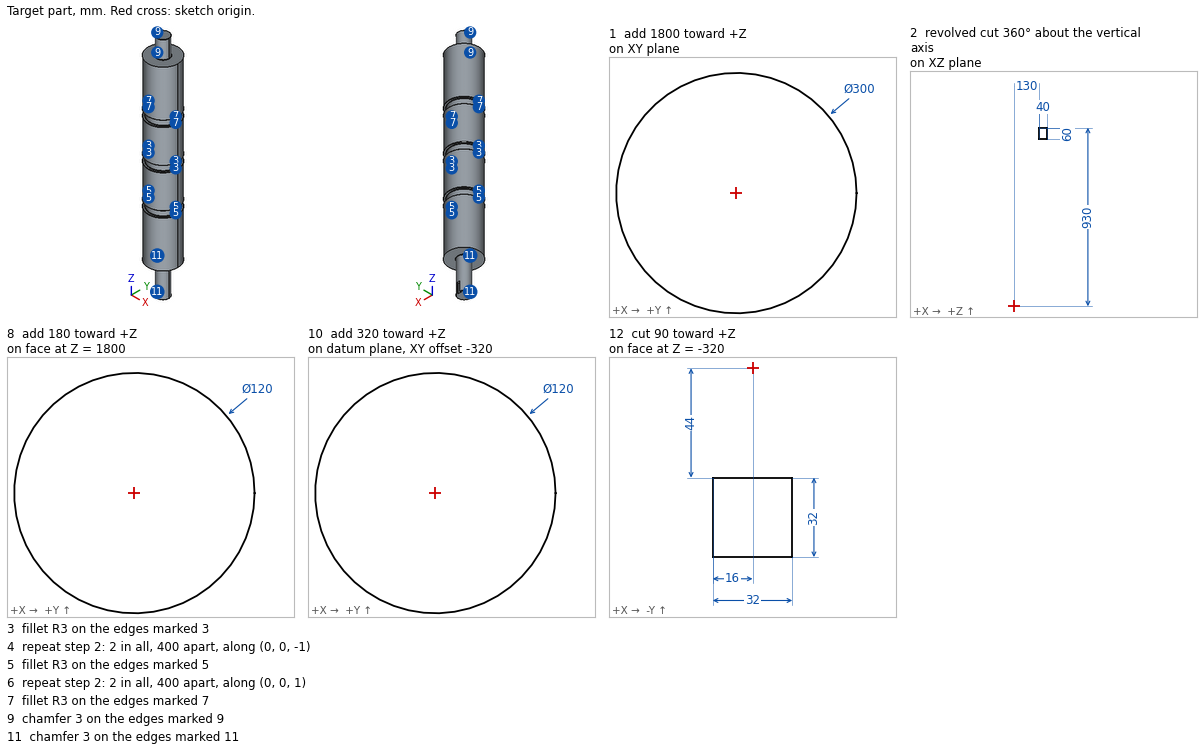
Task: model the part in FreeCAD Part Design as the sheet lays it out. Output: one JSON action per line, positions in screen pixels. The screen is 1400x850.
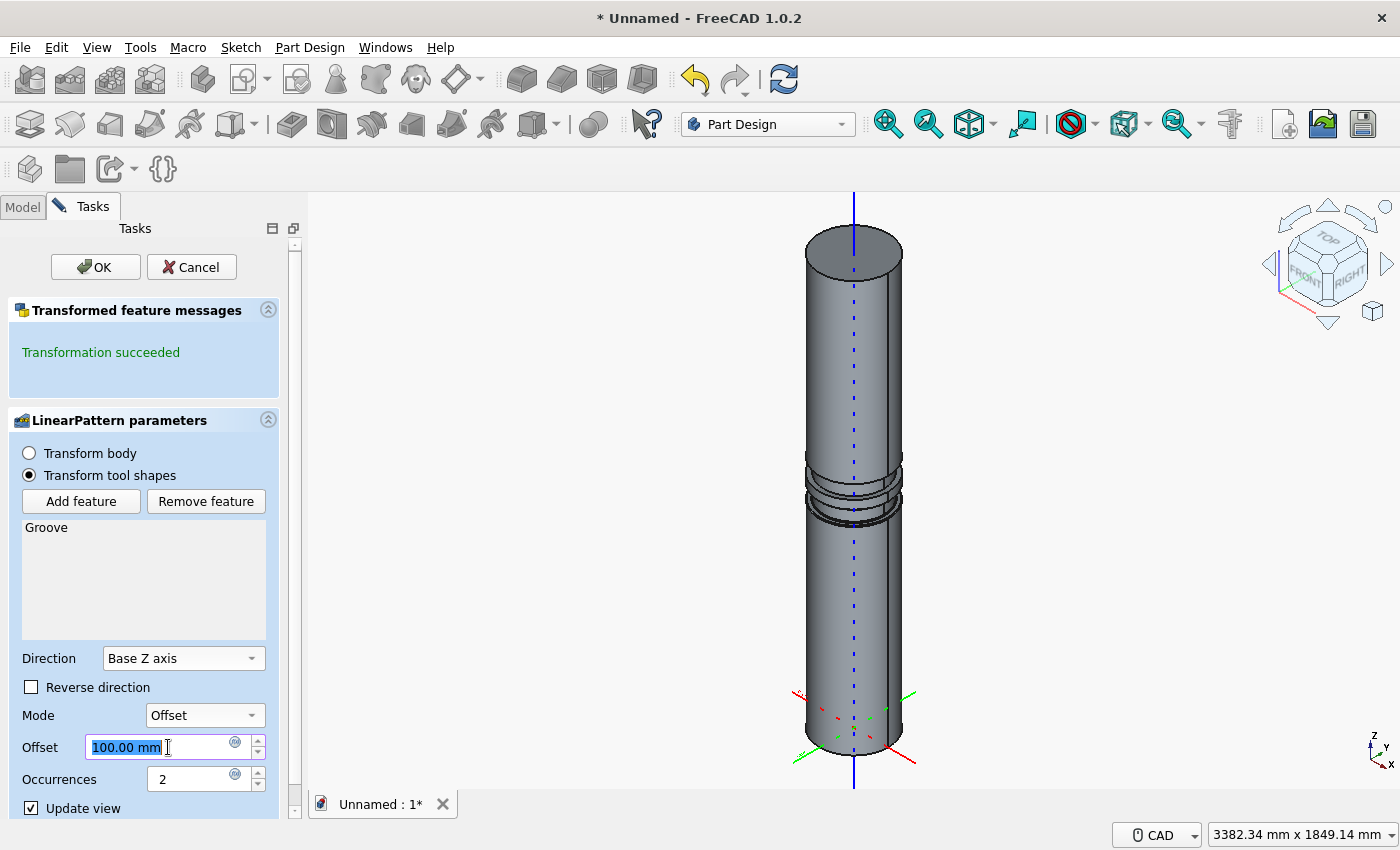
{"action": "type", "text": "400"}
{"action": "key", "text": "Tab"}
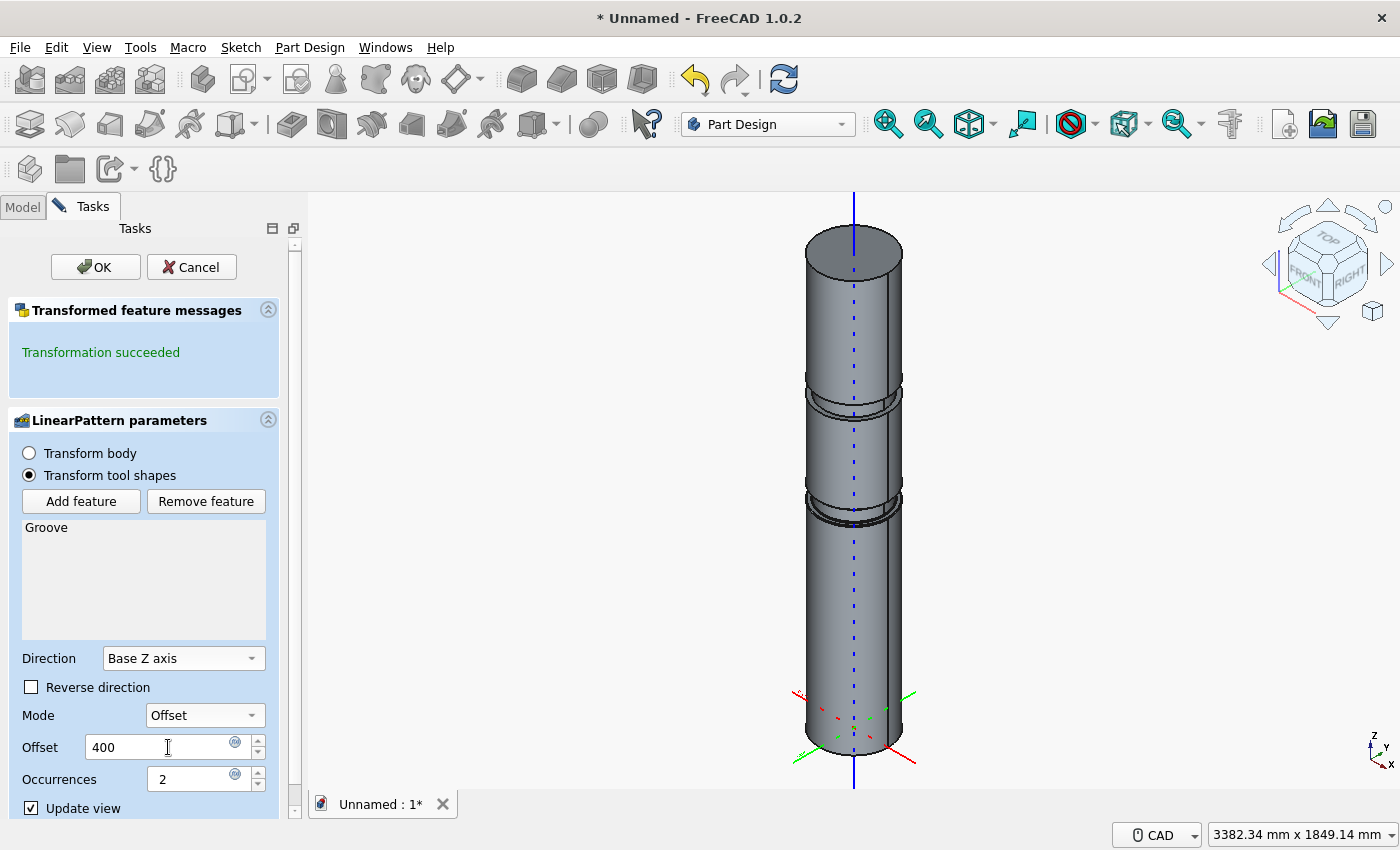
{"action": "triple_click", "coordinate": [198, 779]}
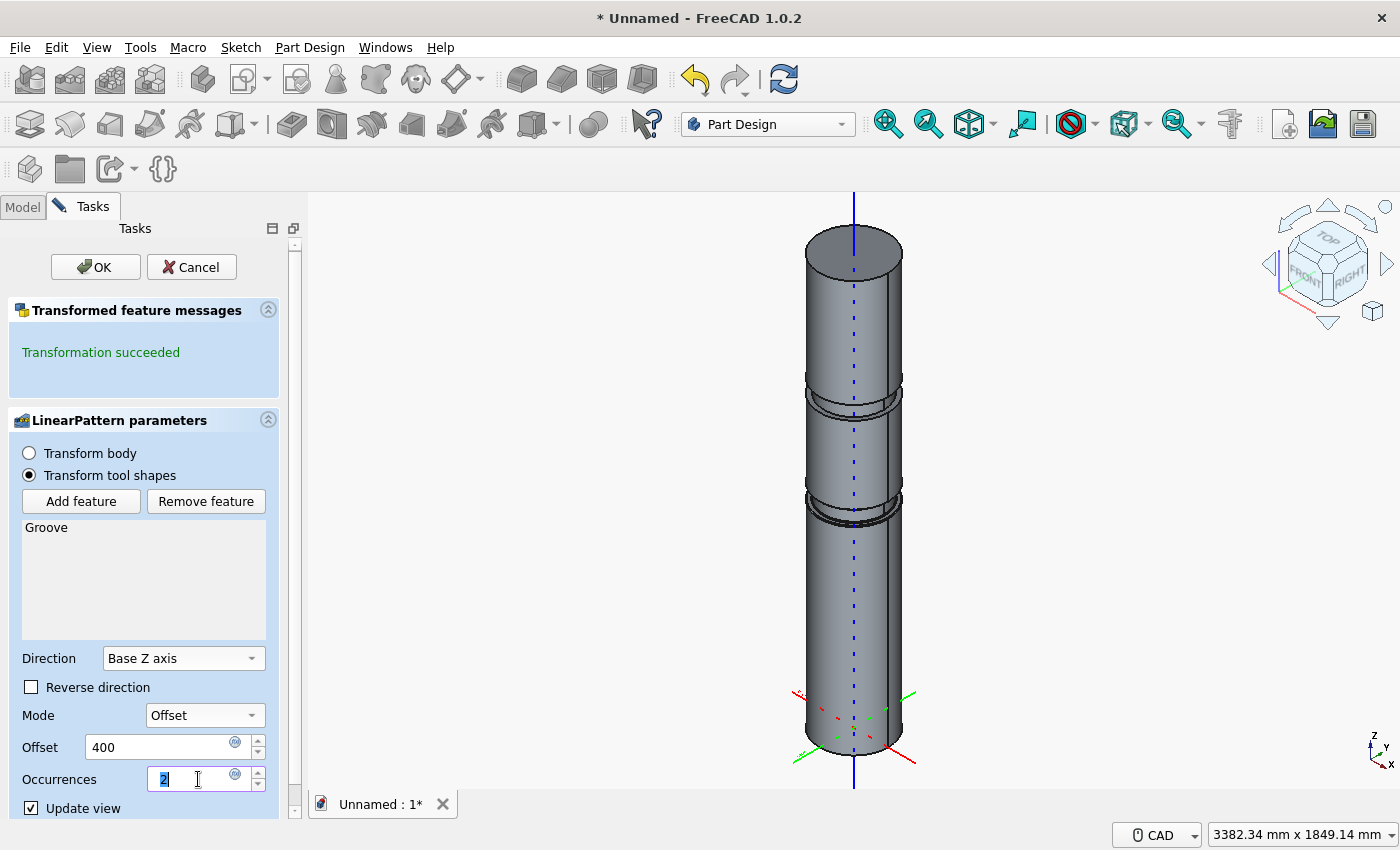
{"action": "type", "text": "2"}
{"action": "key", "text": "Tab"}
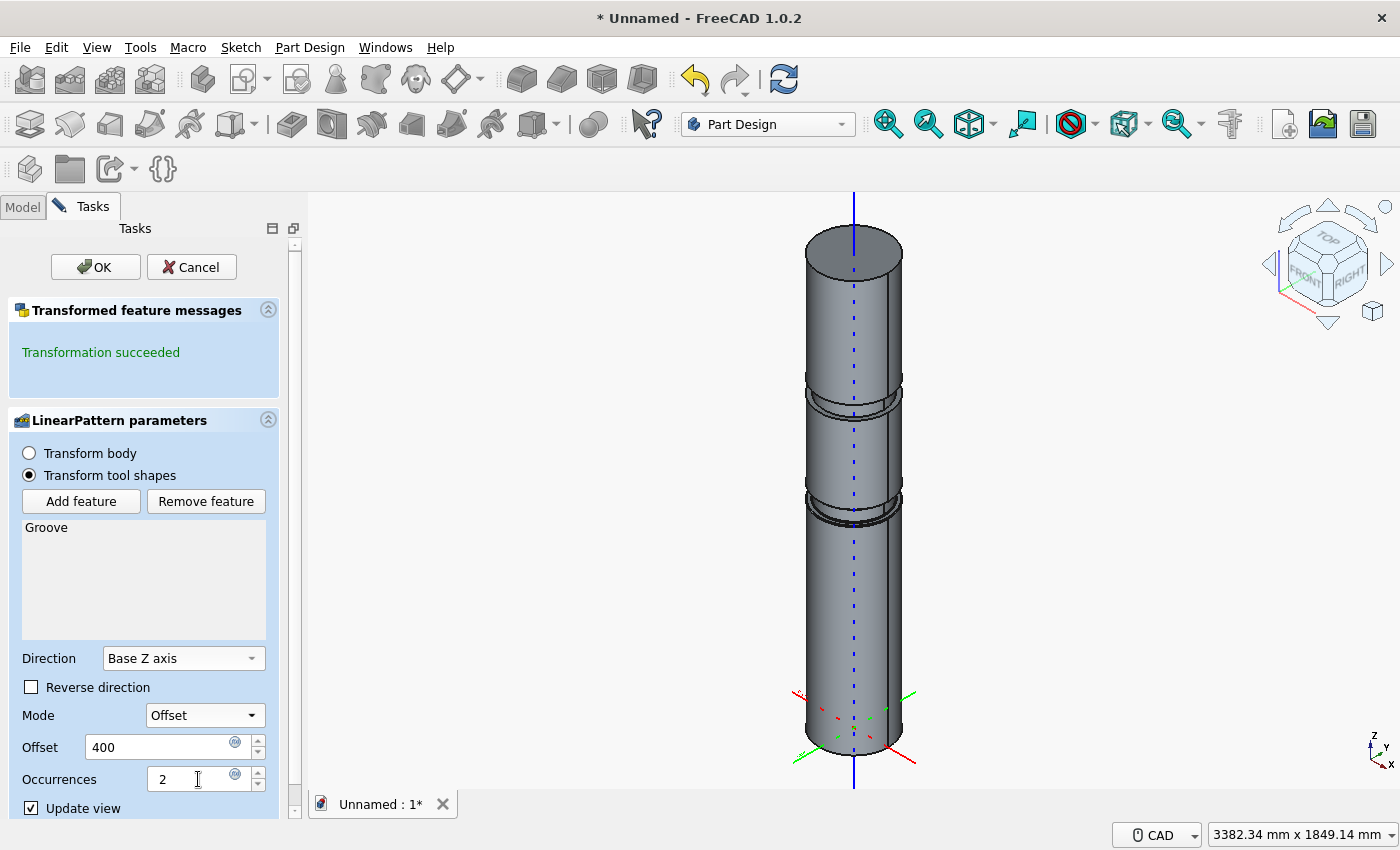
{"action": "left_click", "coordinate": [30, 687]}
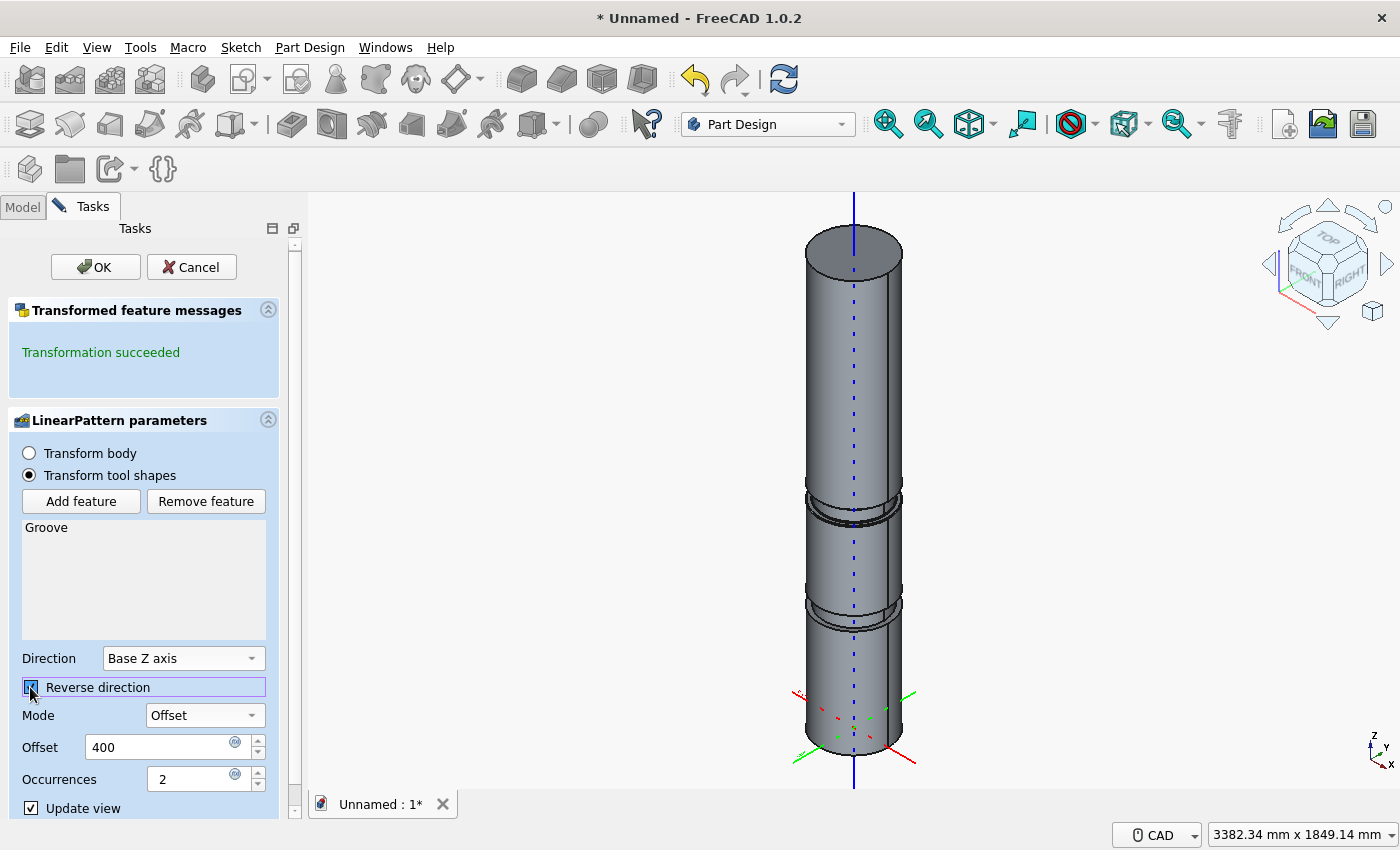
{"action": "left_click", "coordinate": [96, 267]}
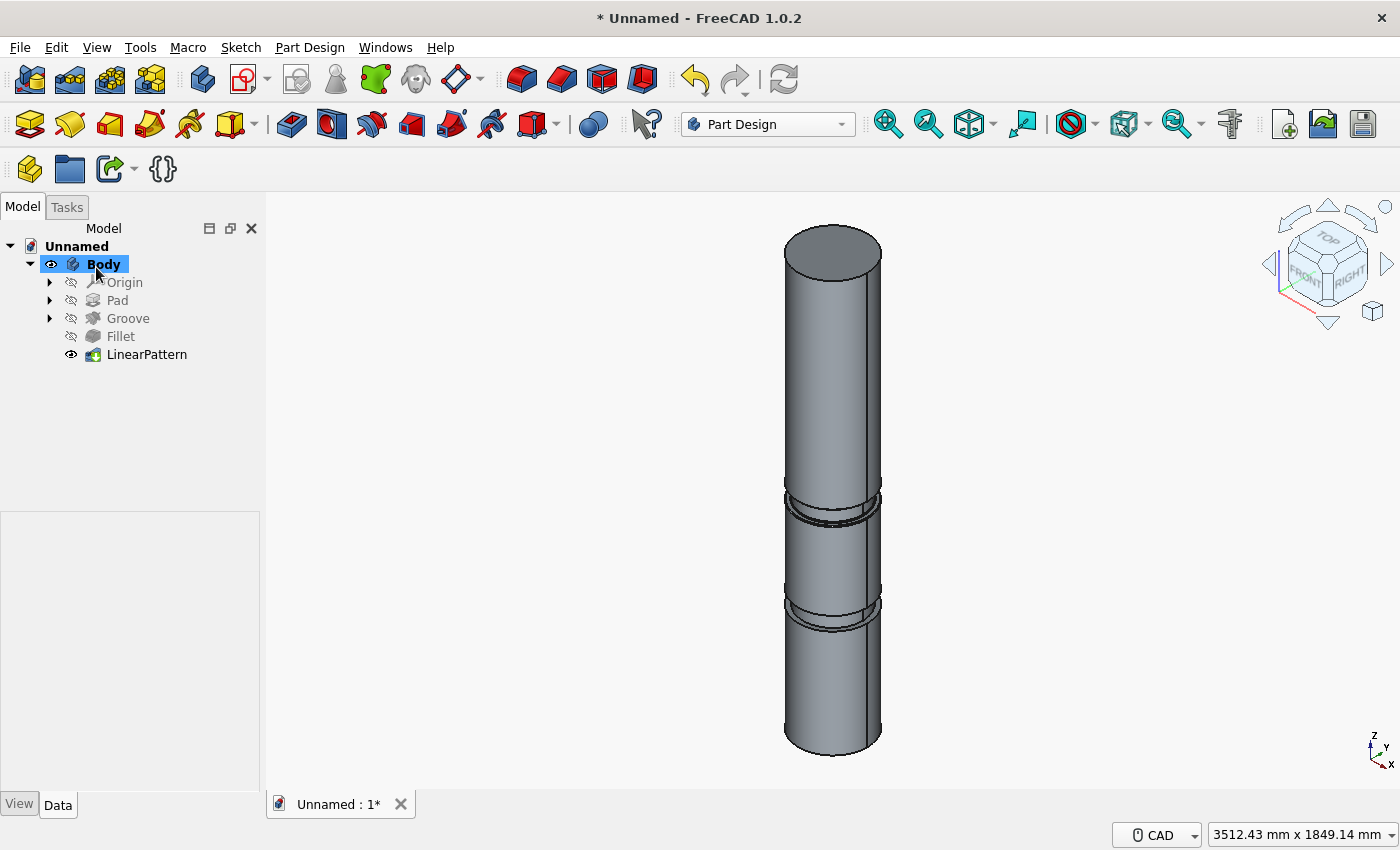
{"action": "left_click", "coordinate": [790, 615]}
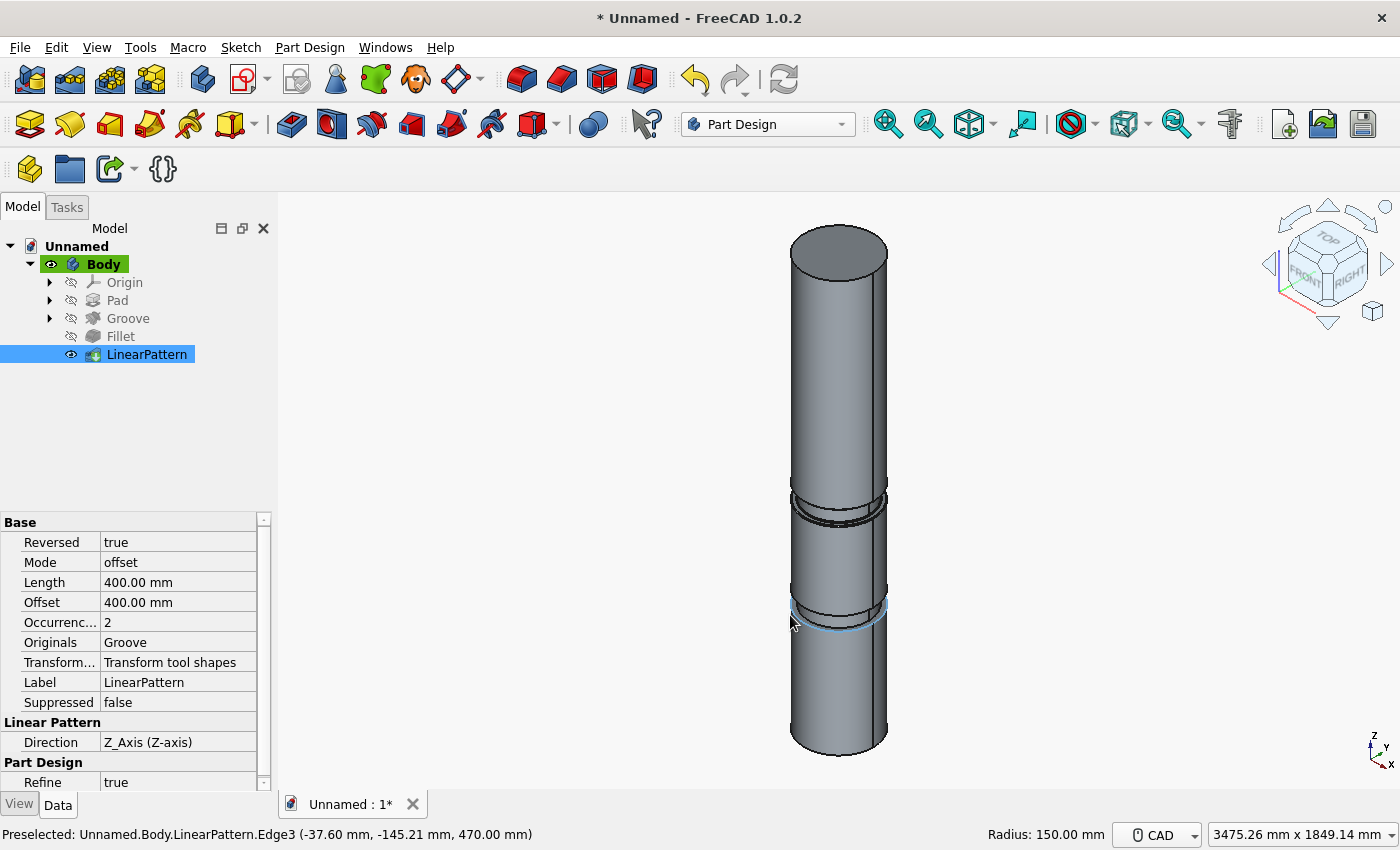
{"action": "key", "text": "2"}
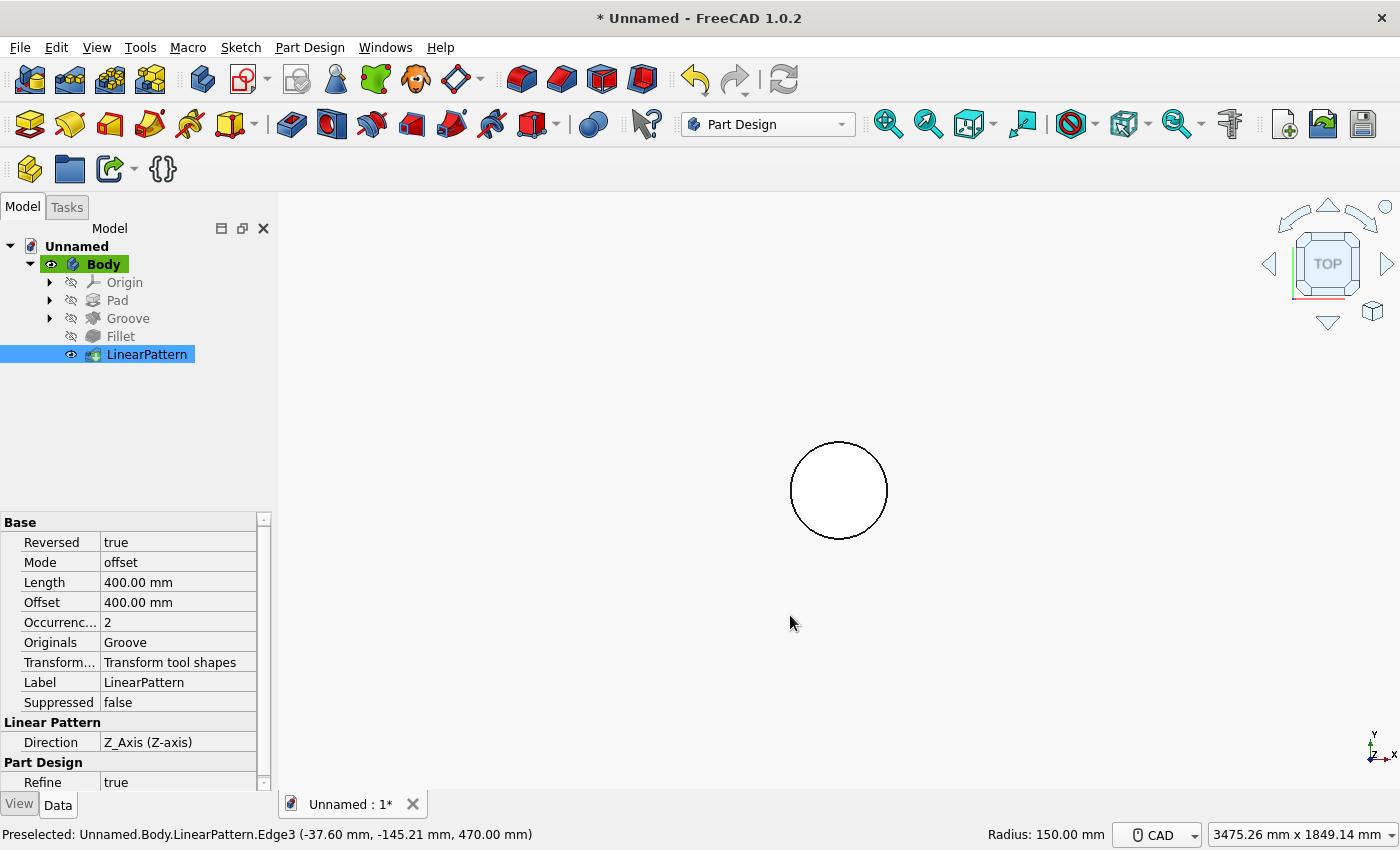
{"action": "left_click", "coordinate": [890, 124]}